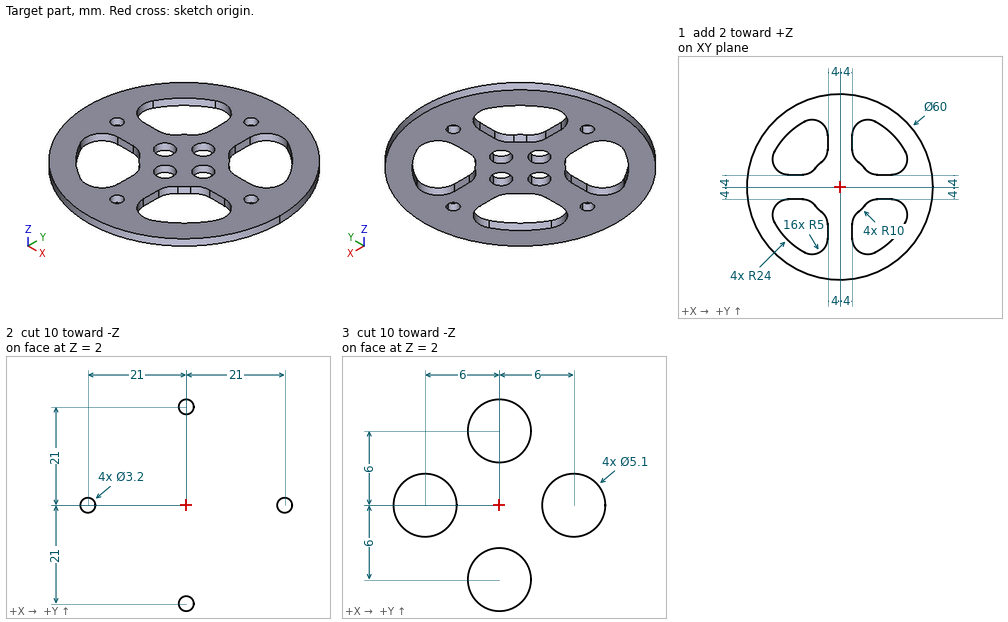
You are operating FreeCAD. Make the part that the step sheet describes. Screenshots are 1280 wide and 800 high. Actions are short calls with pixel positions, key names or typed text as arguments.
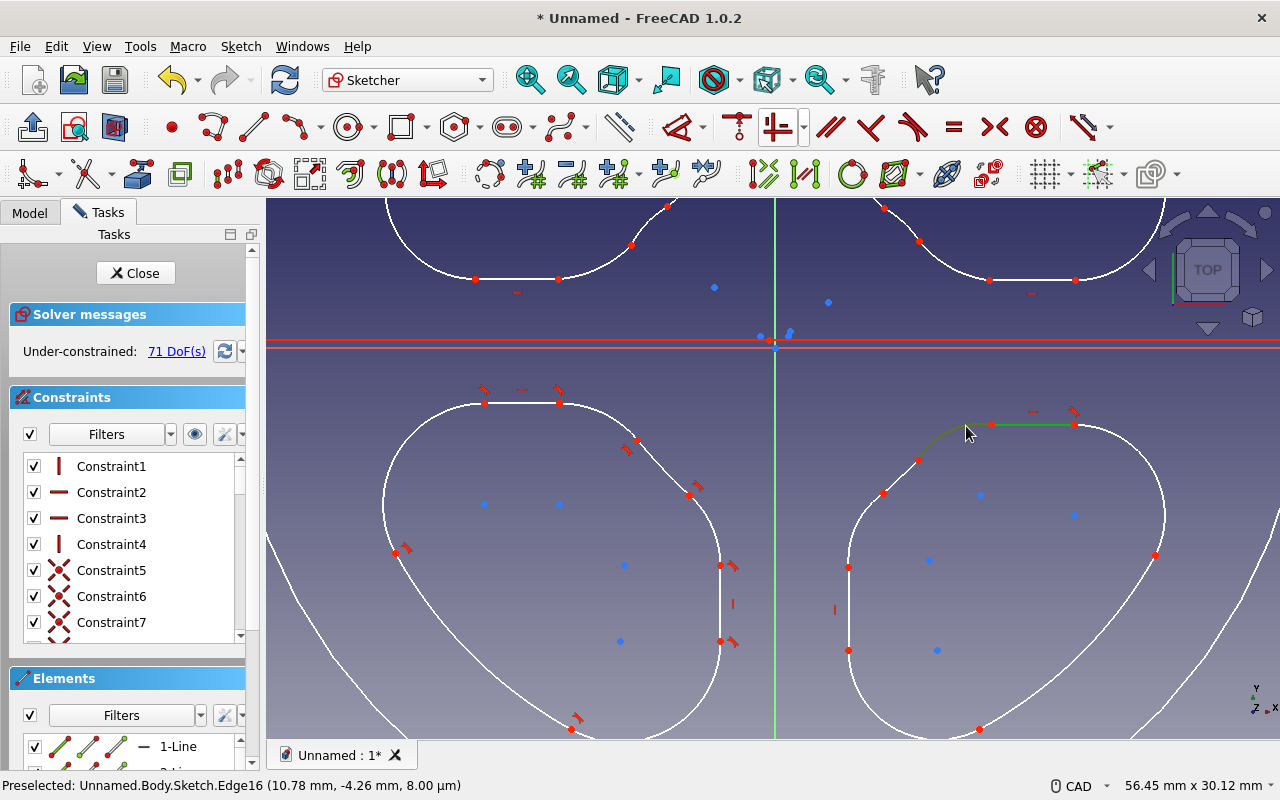
key(t)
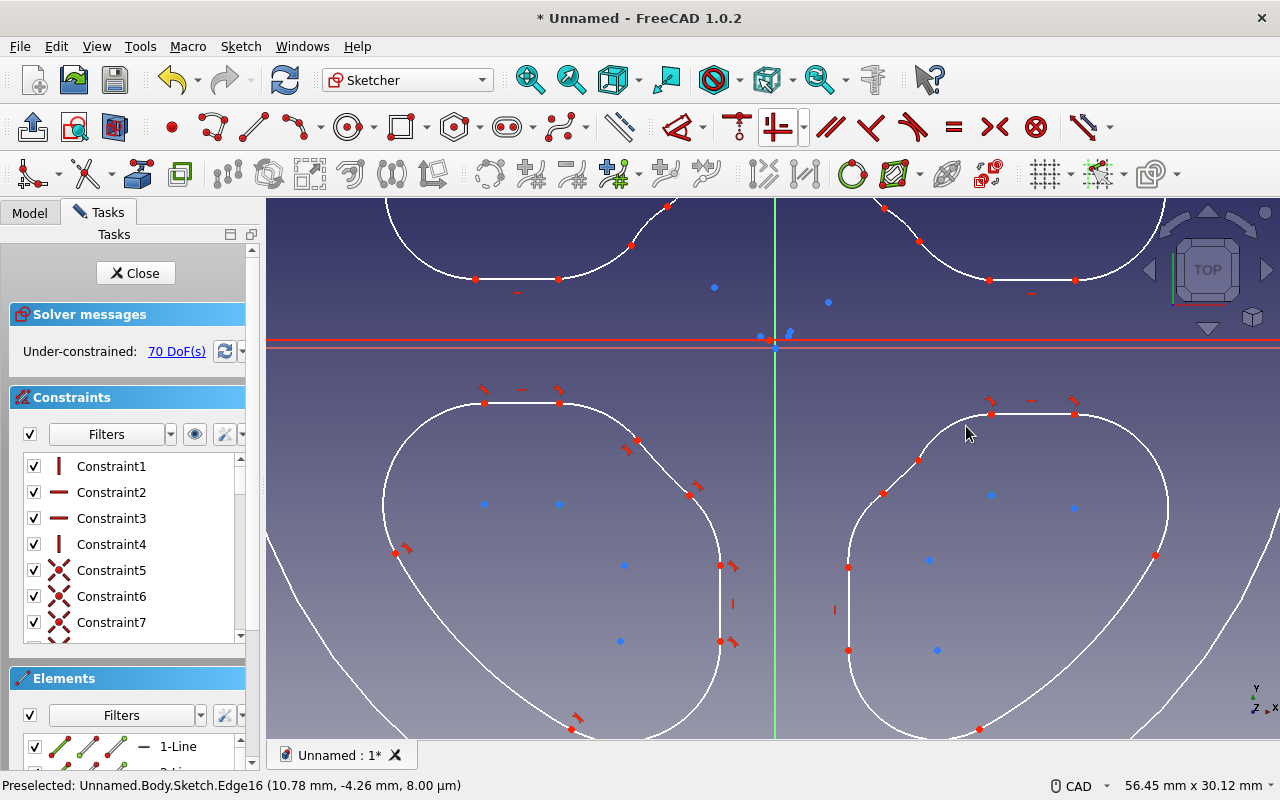
click(849, 626)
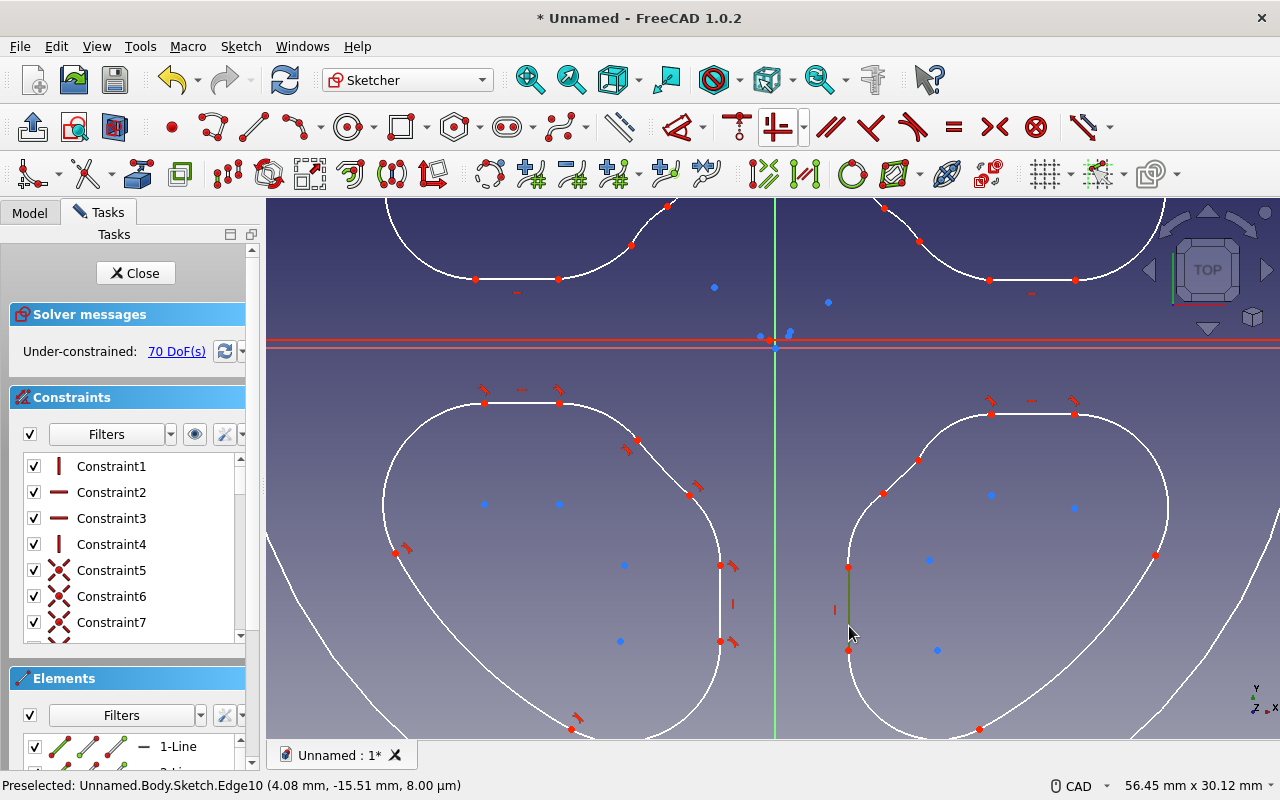
click(865, 702)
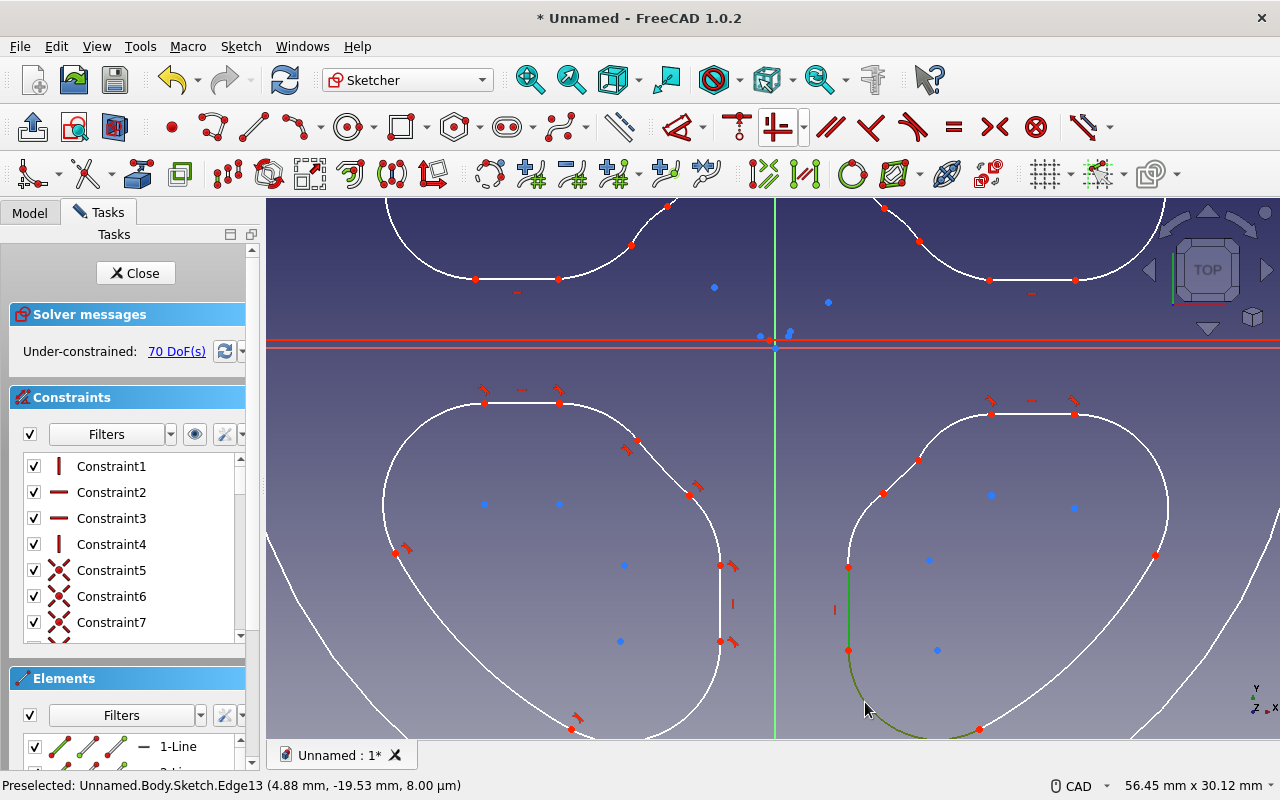
click(913, 128)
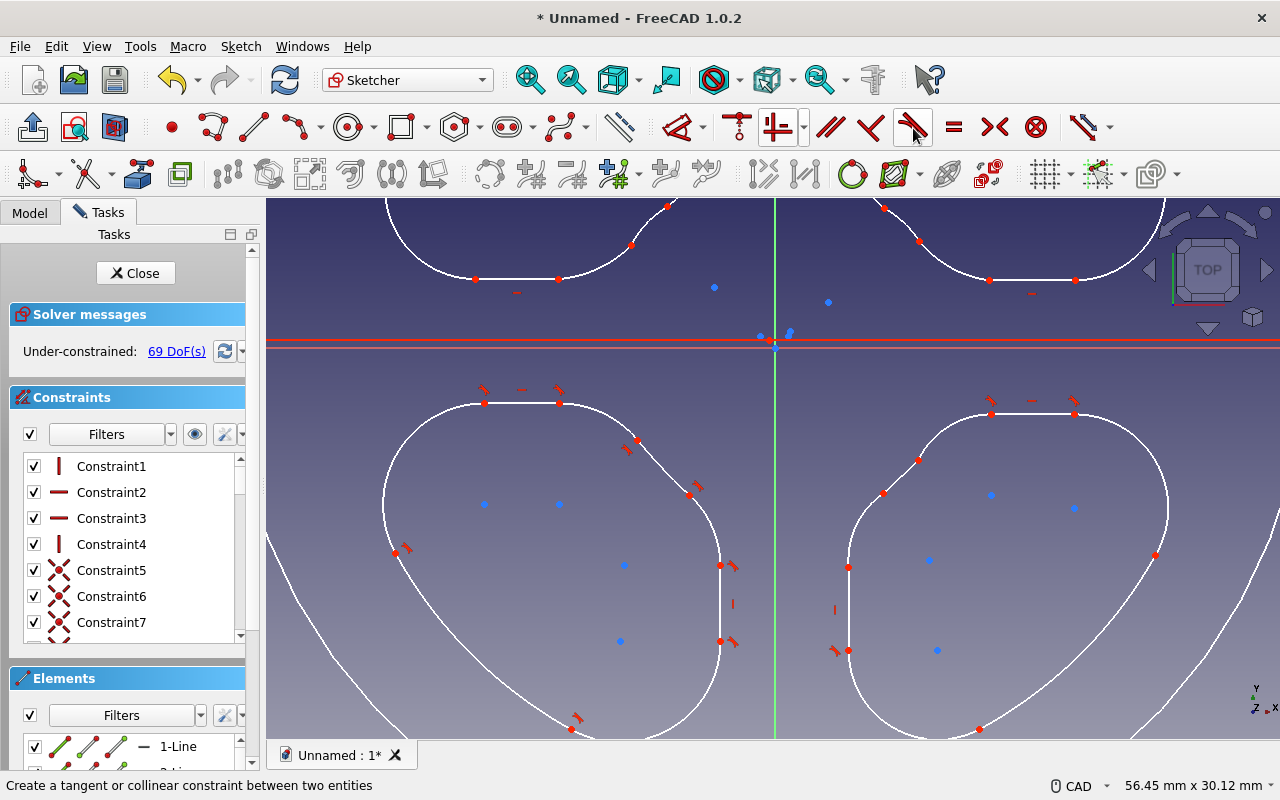
click(849, 626)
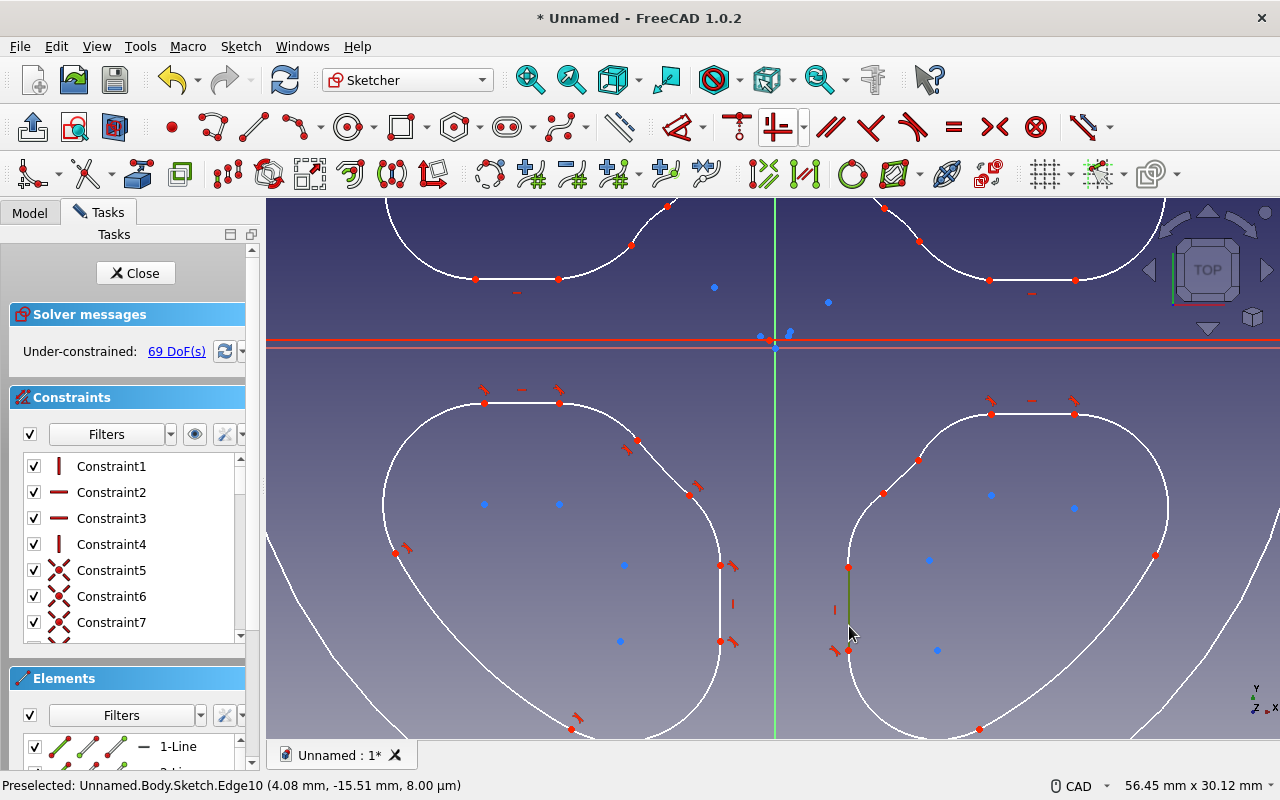
click(865, 511)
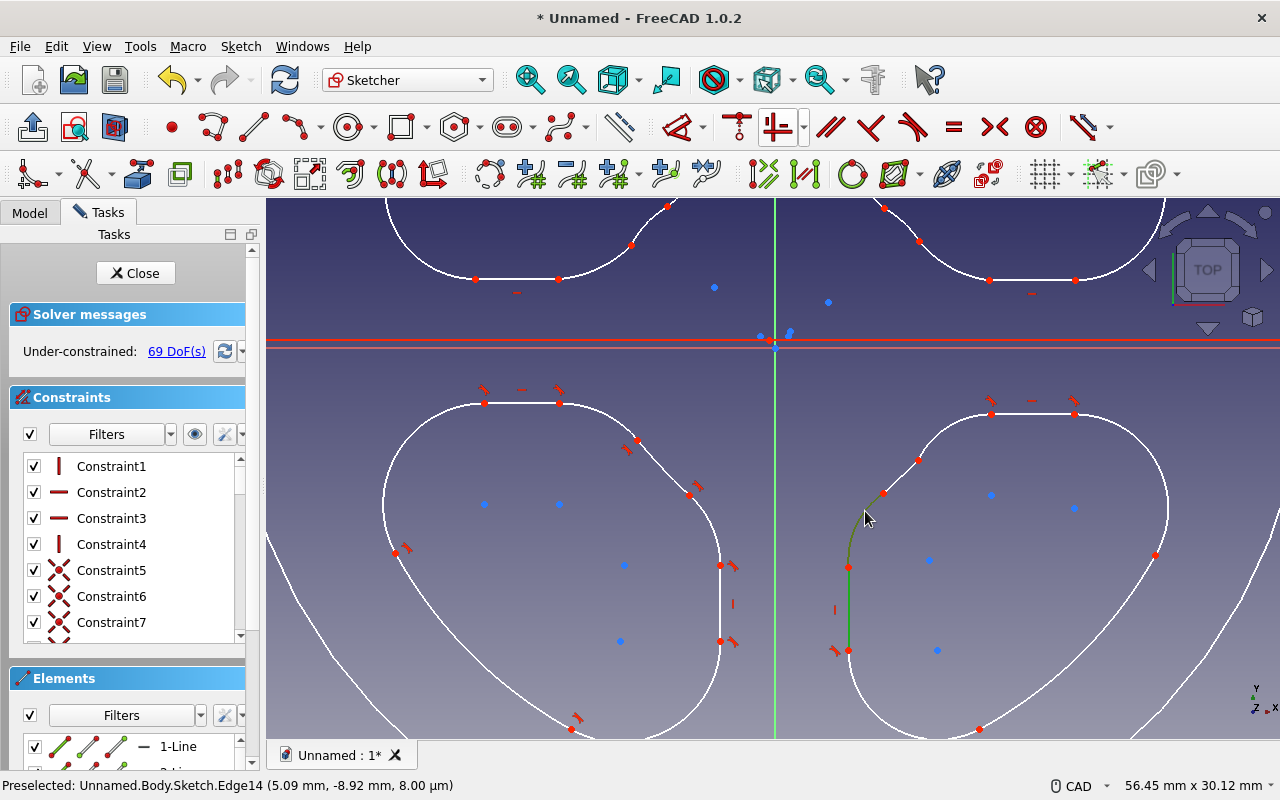
click(913, 128)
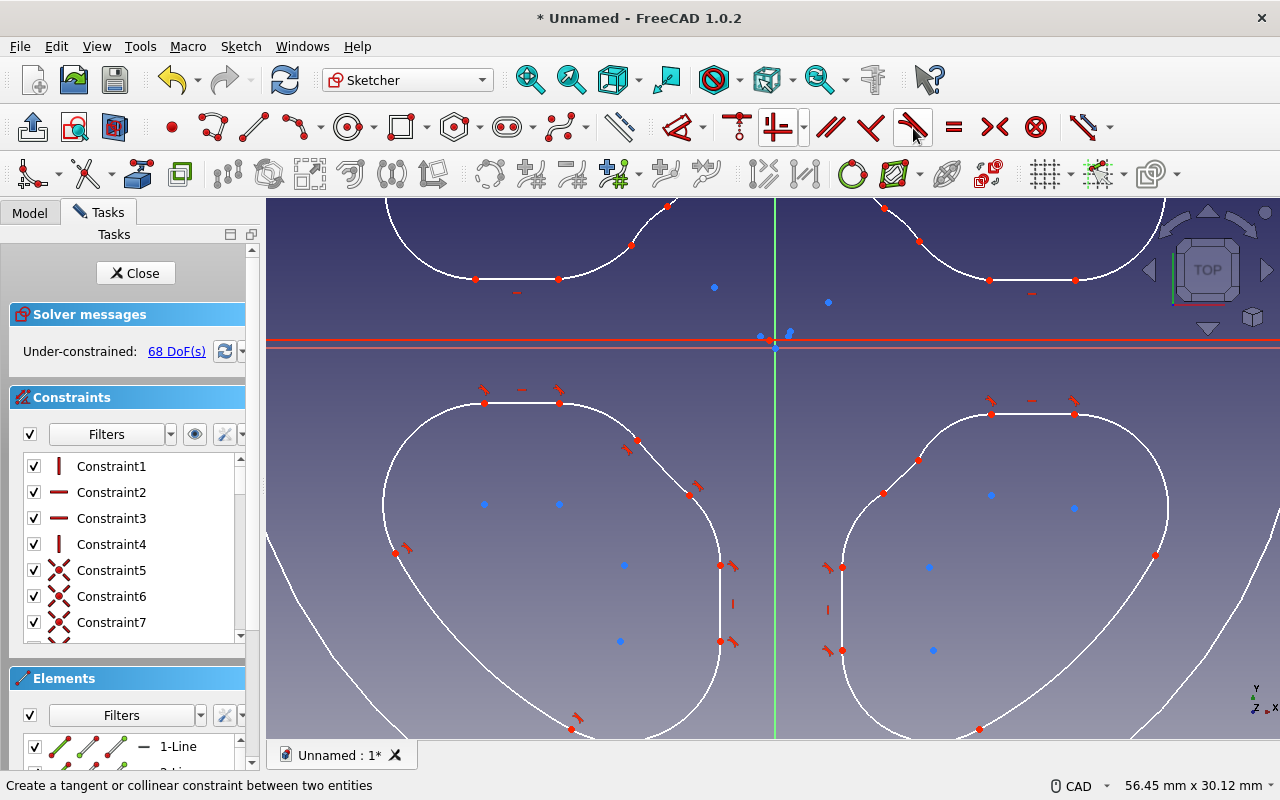
click(1113, 423)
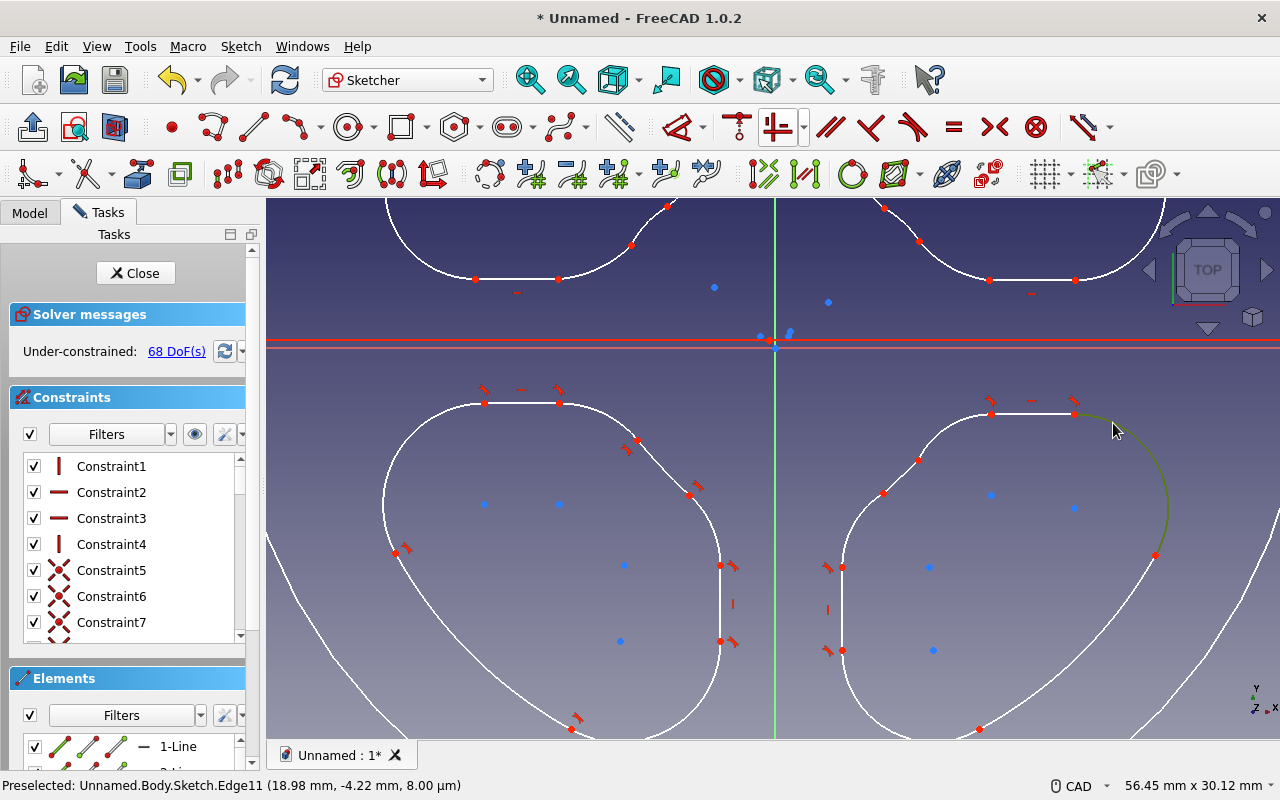
click(1042, 688)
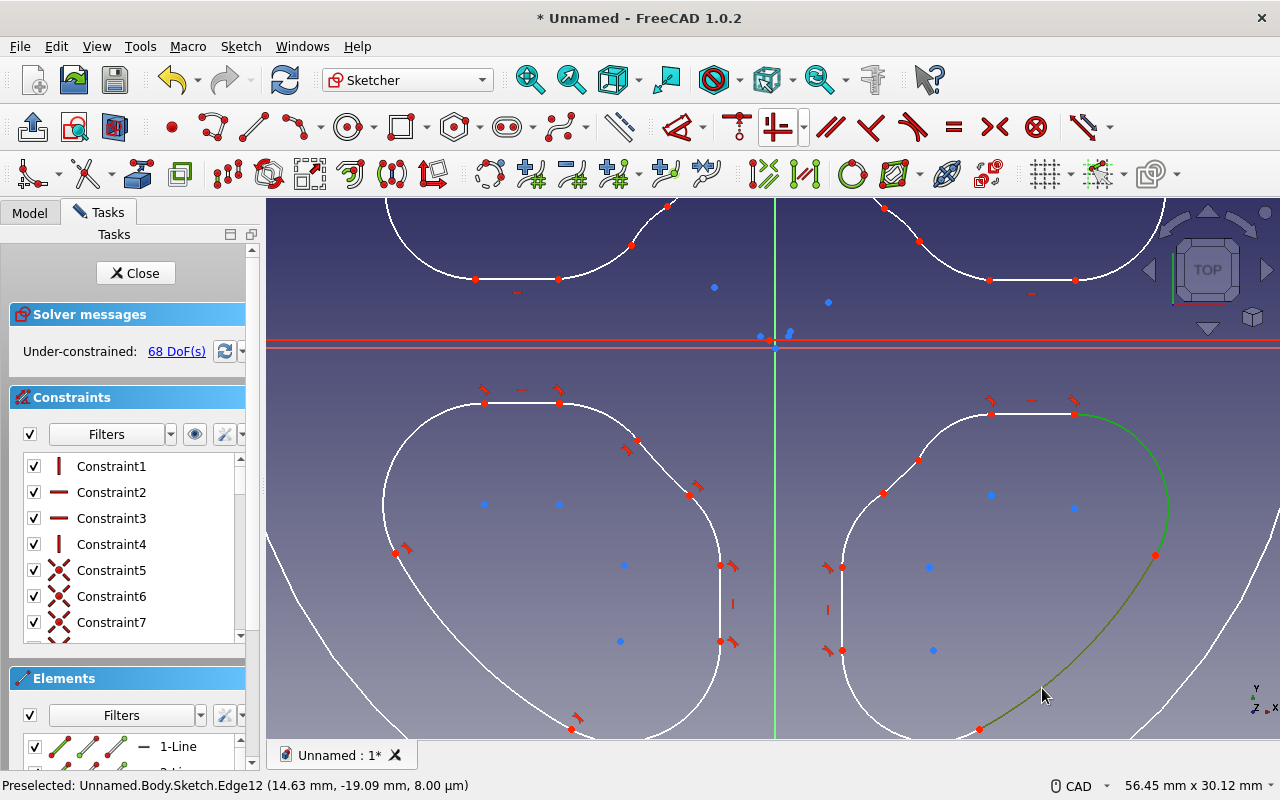
key(t)